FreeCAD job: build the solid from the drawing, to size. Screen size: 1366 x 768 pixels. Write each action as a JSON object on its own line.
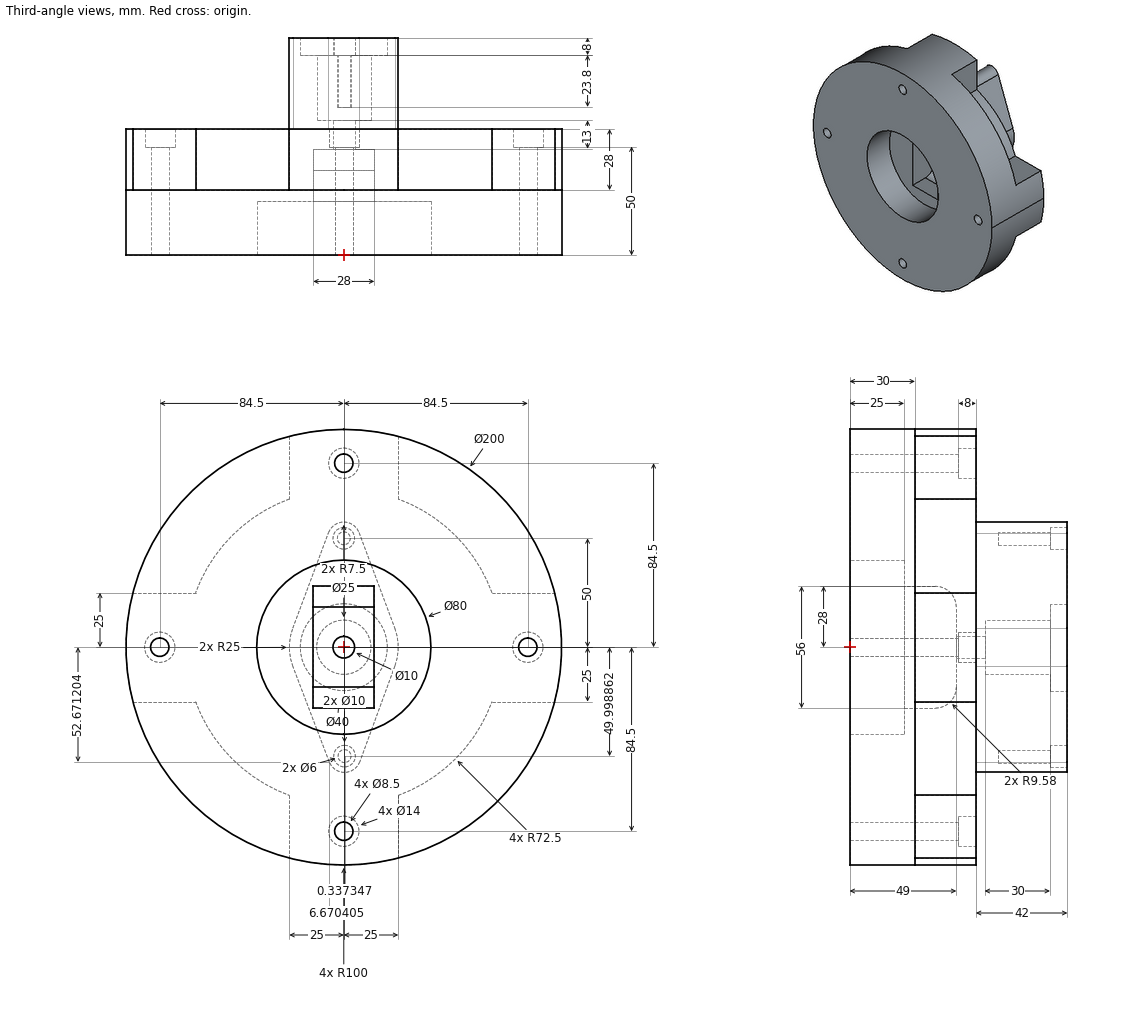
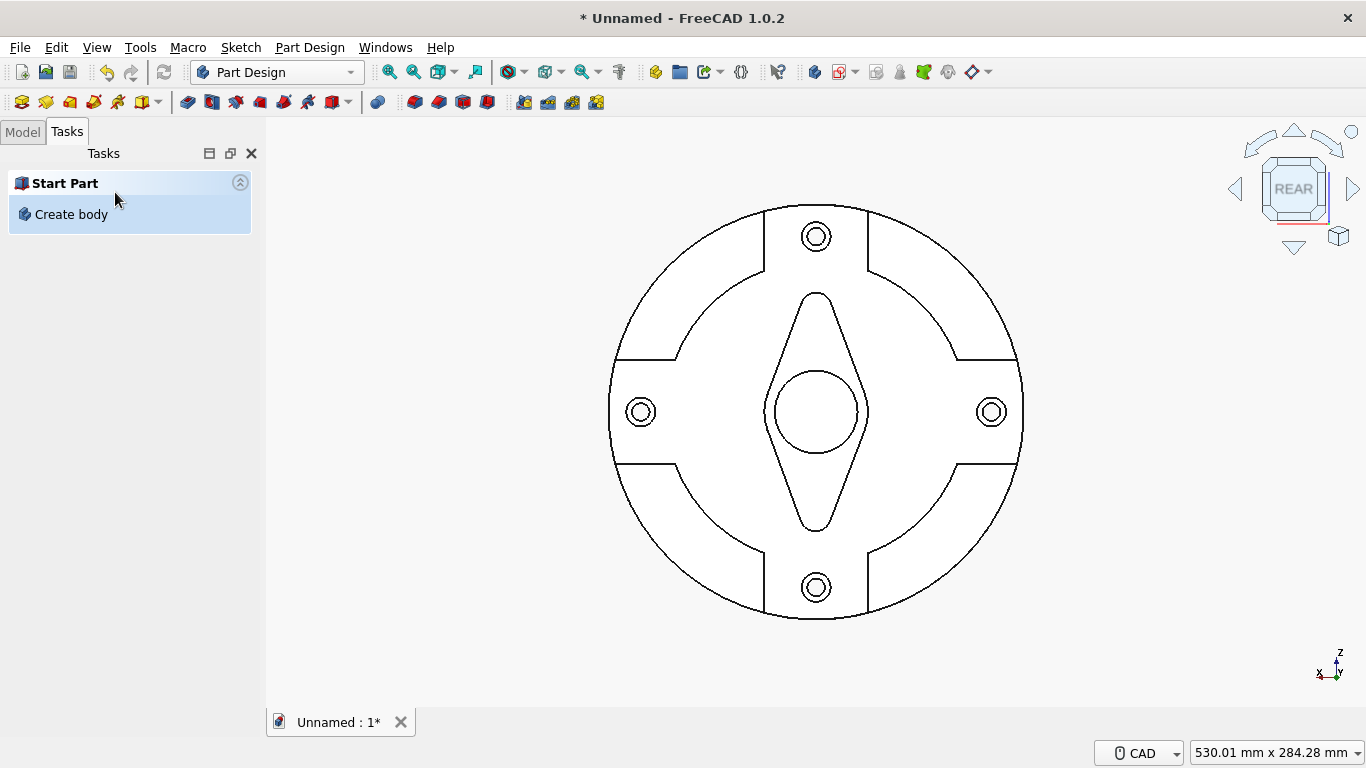
{"action": "left_click", "coordinate": [816, 411]}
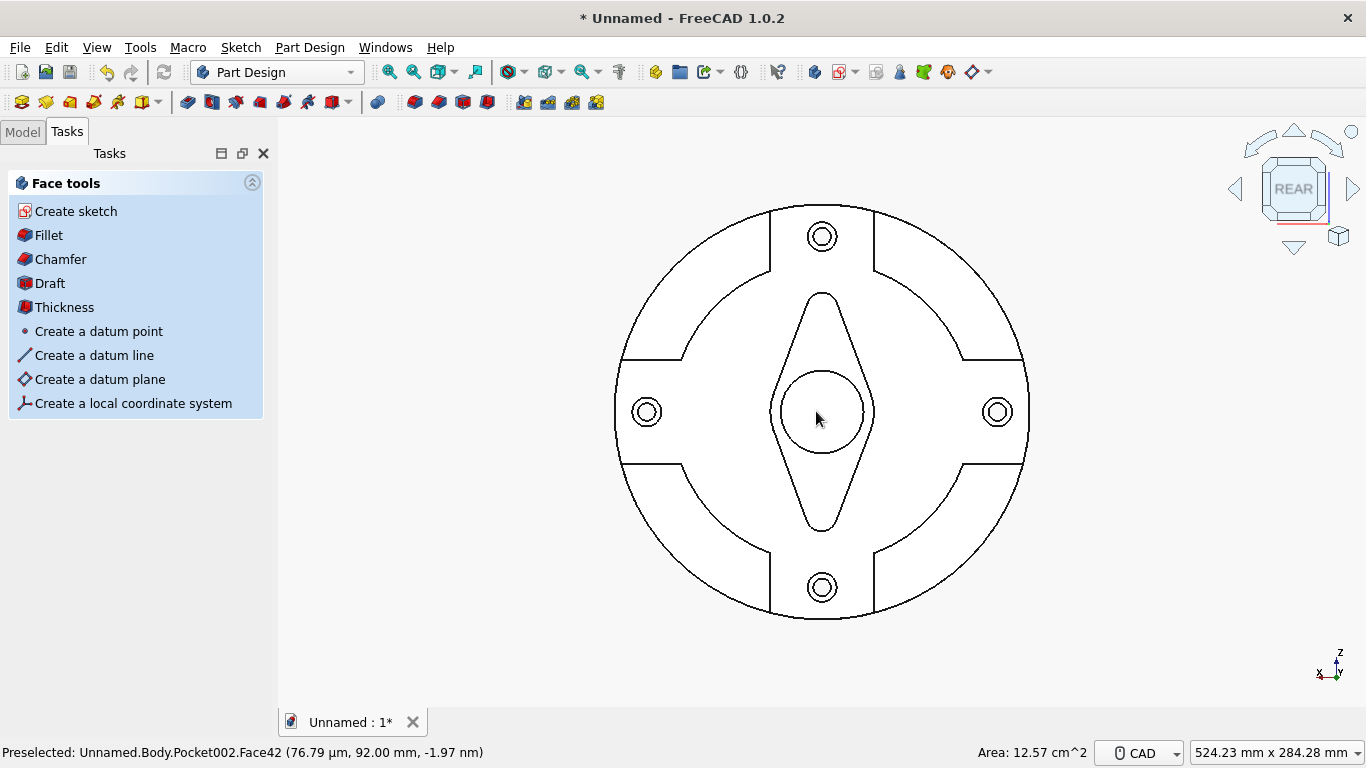
{"action": "left_click", "coordinate": [840, 72]}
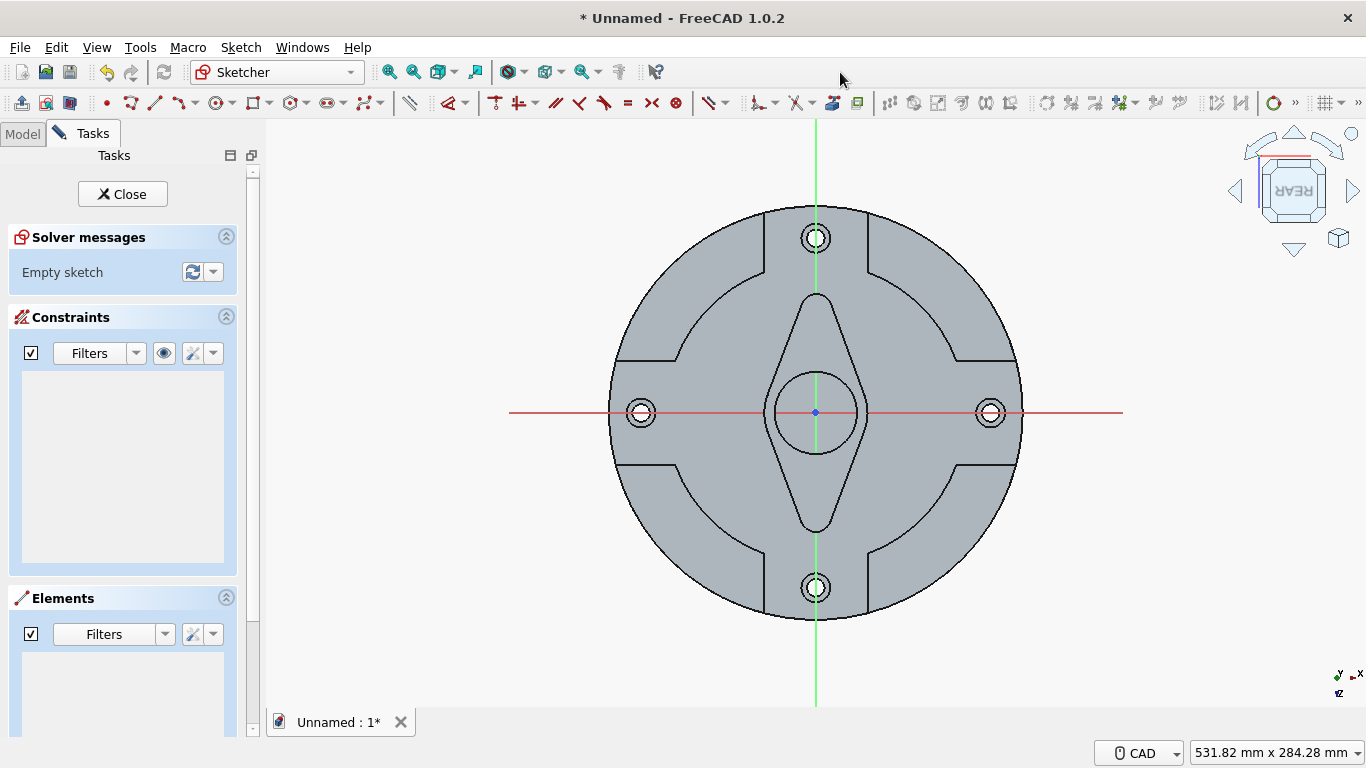
{"action": "scroll", "coordinate": [827, 413], "scroll_direction": "up", "scroll_amount": 10}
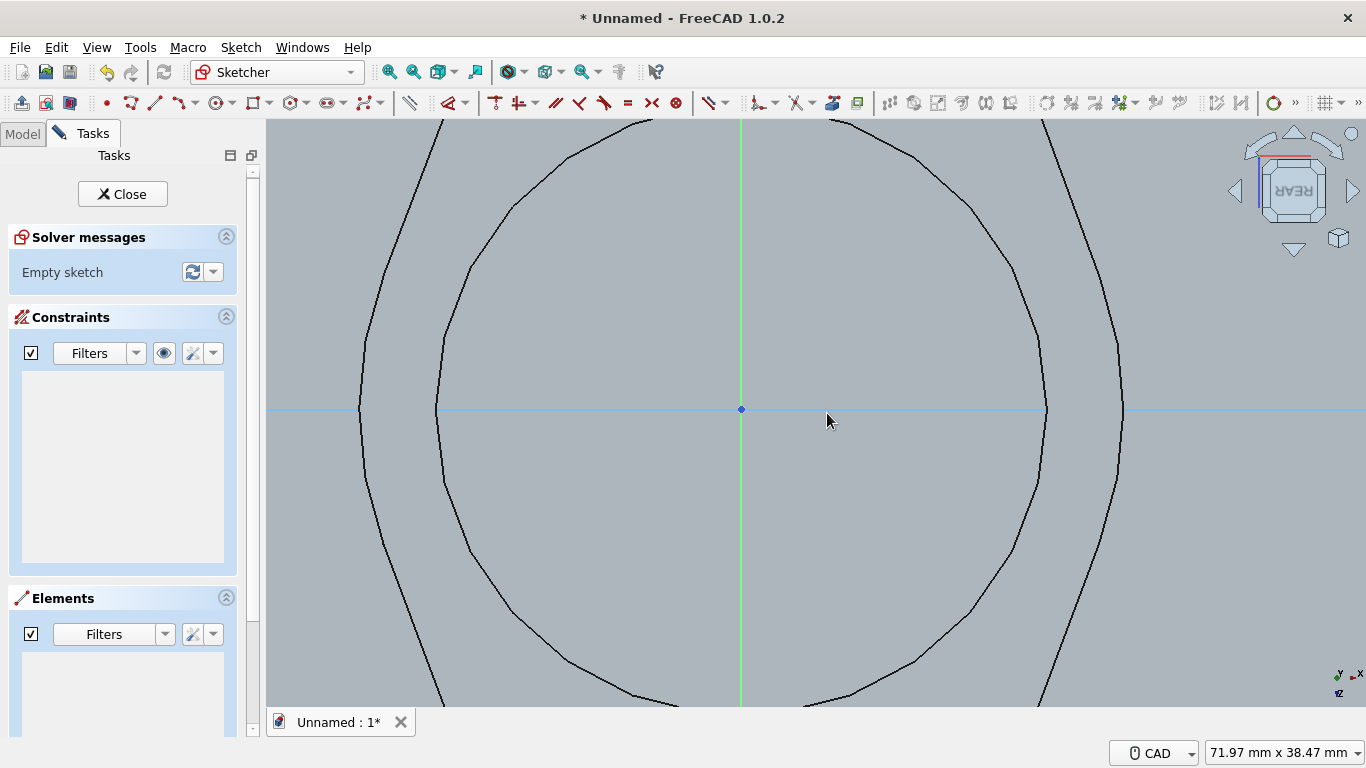
{"action": "key", "text": "g c"}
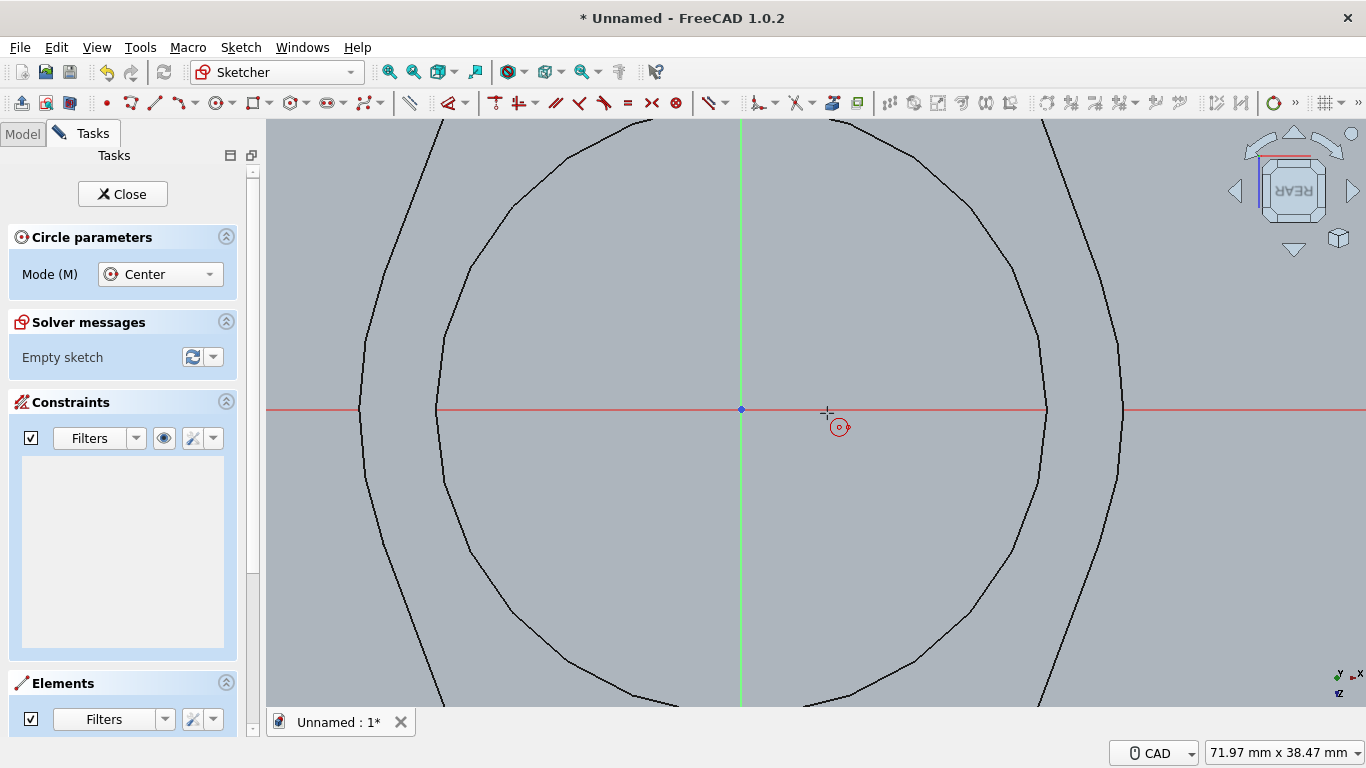
{"action": "left_click", "coordinate": [741, 410]}
{"action": "left_click", "coordinate": [876, 275]}
{"action": "key", "text": "Escape"}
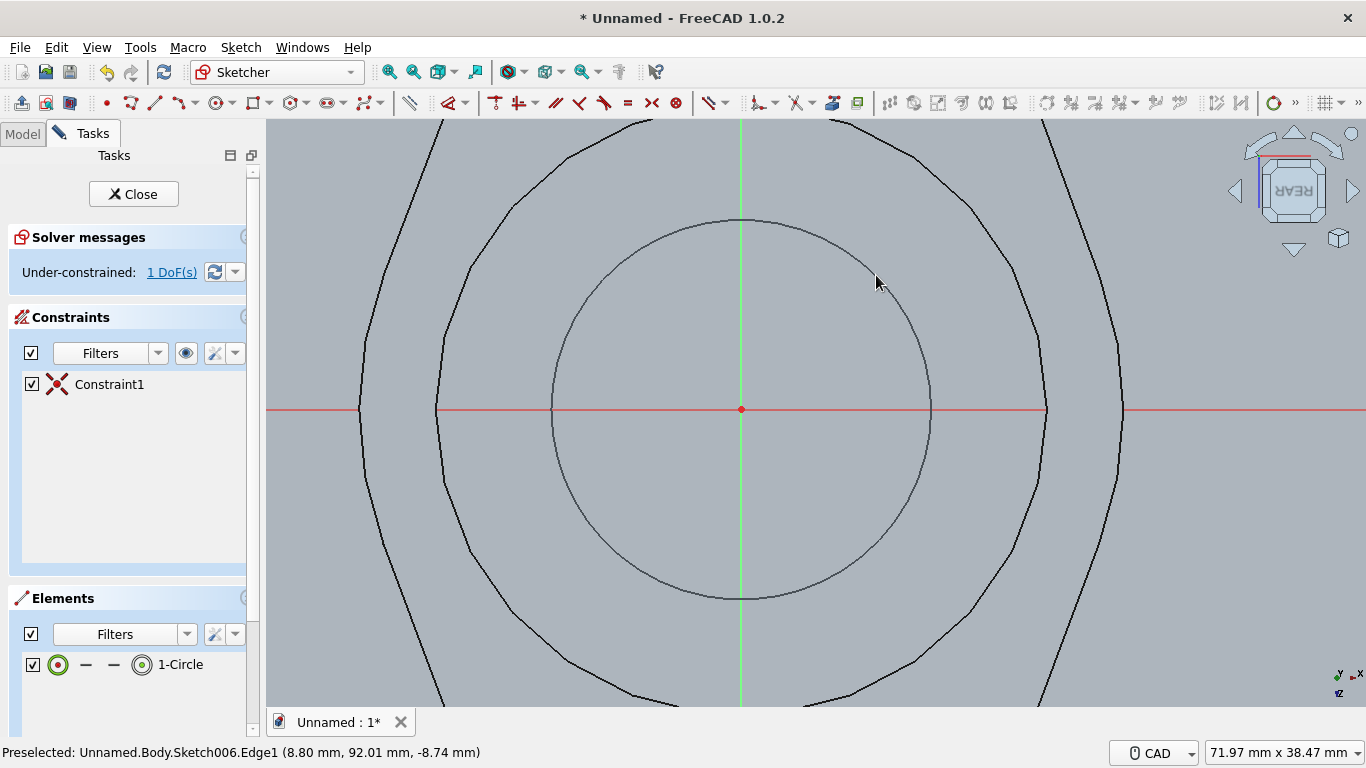
{"action": "left_click", "coordinate": [448, 104]}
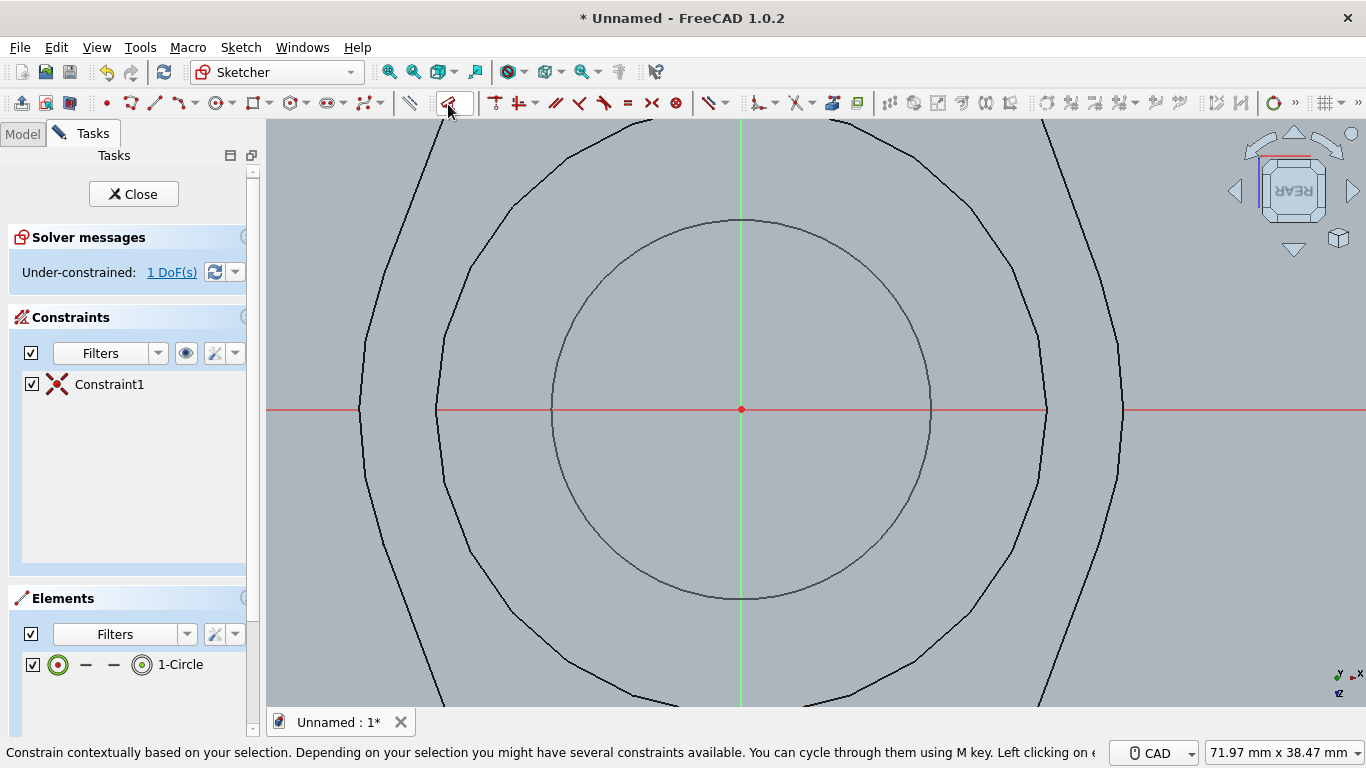
{"action": "left_click", "coordinate": [875, 275]}
{"action": "left_click", "coordinate": [898, 252]}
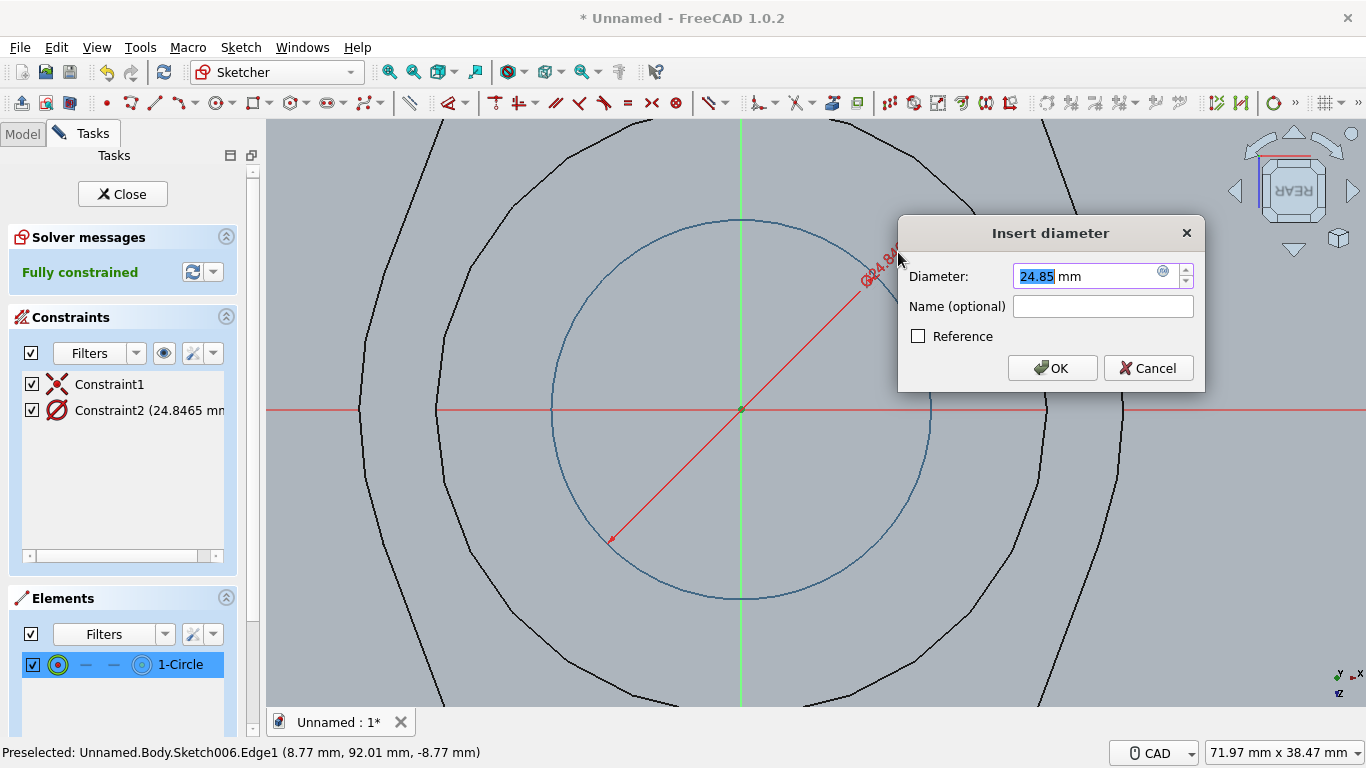
{"action": "type", "text": "25"}
{"action": "key", "text": "Return"}
{"action": "key", "text": "Escape"}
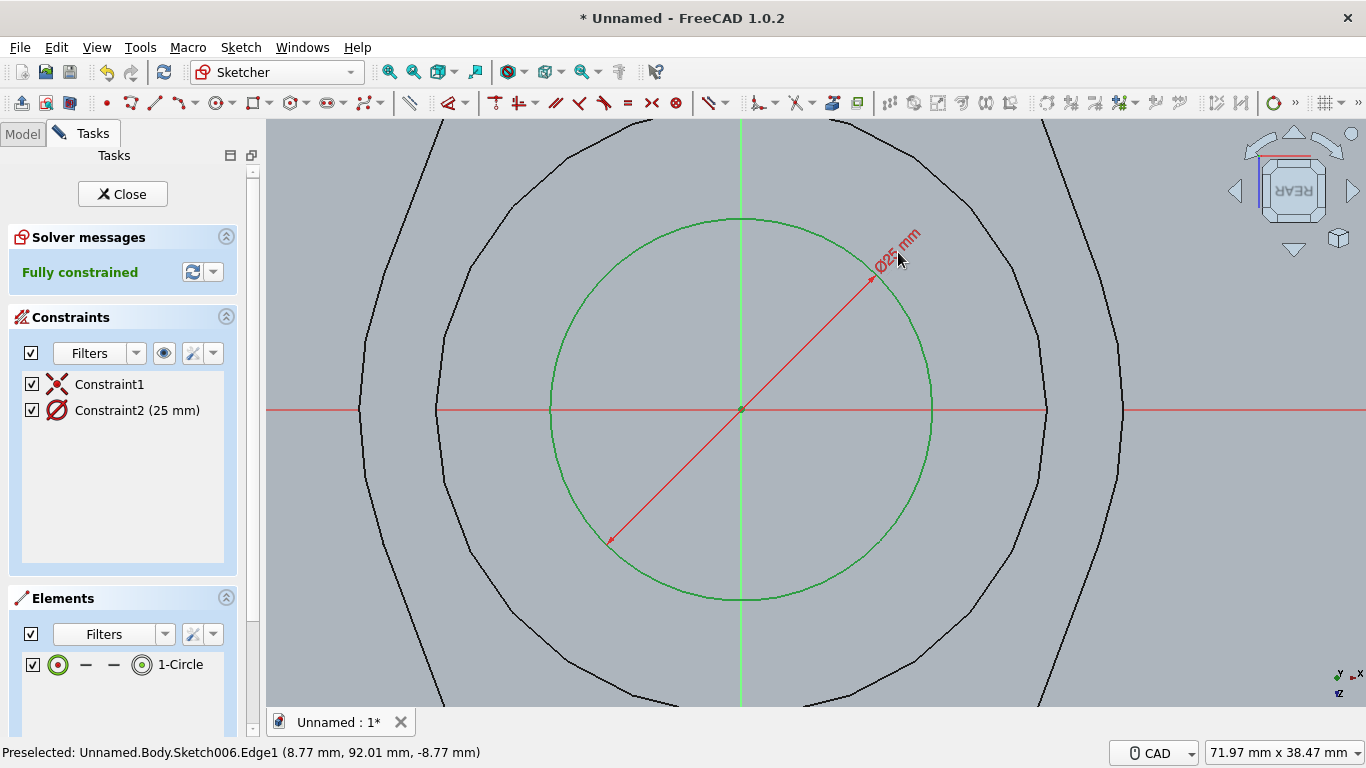
{"action": "left_click", "coordinate": [123, 194]}